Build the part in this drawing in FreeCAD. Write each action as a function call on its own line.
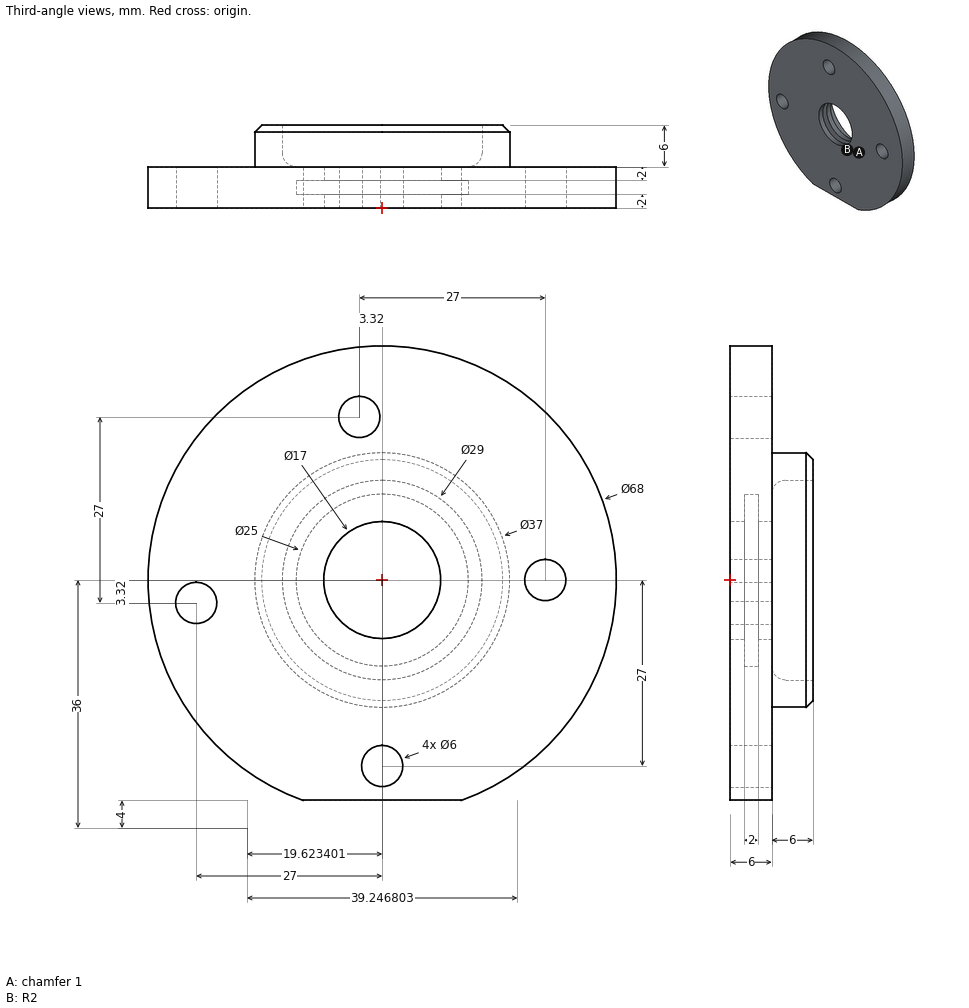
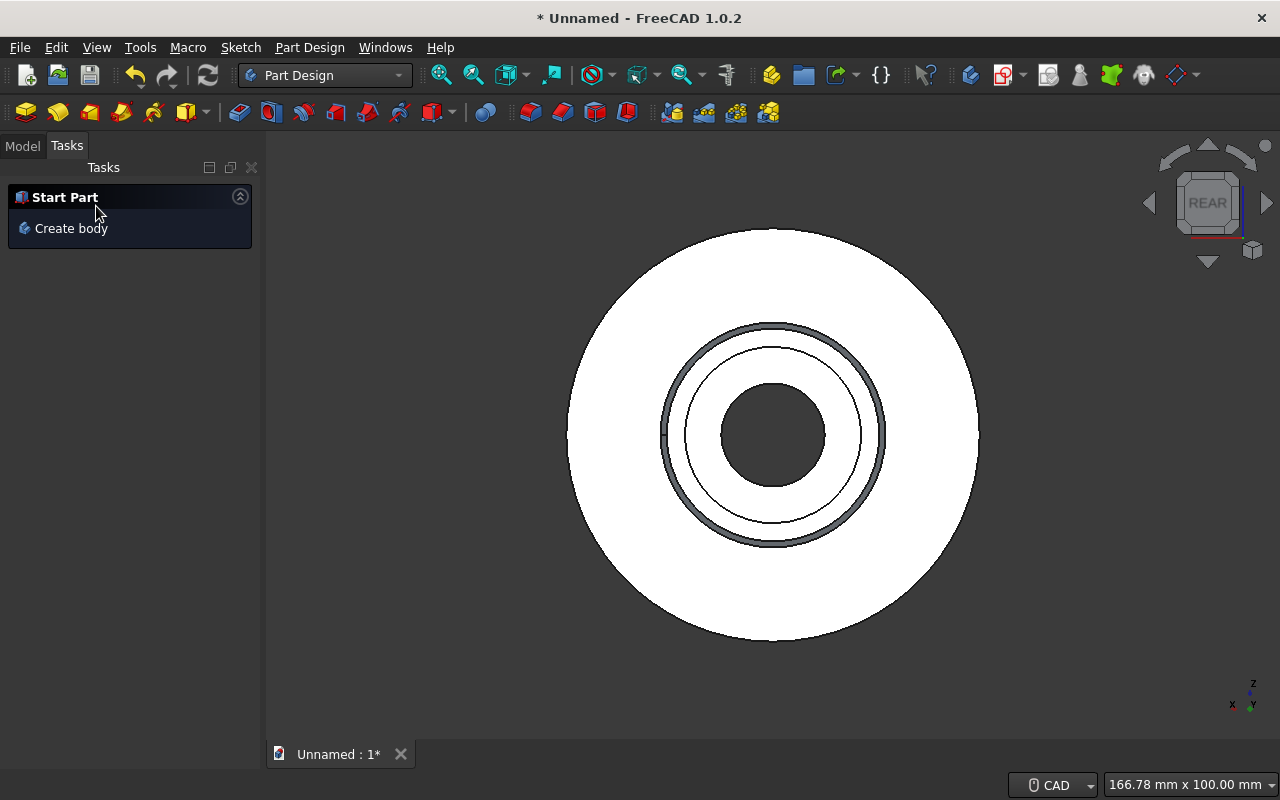
key(0)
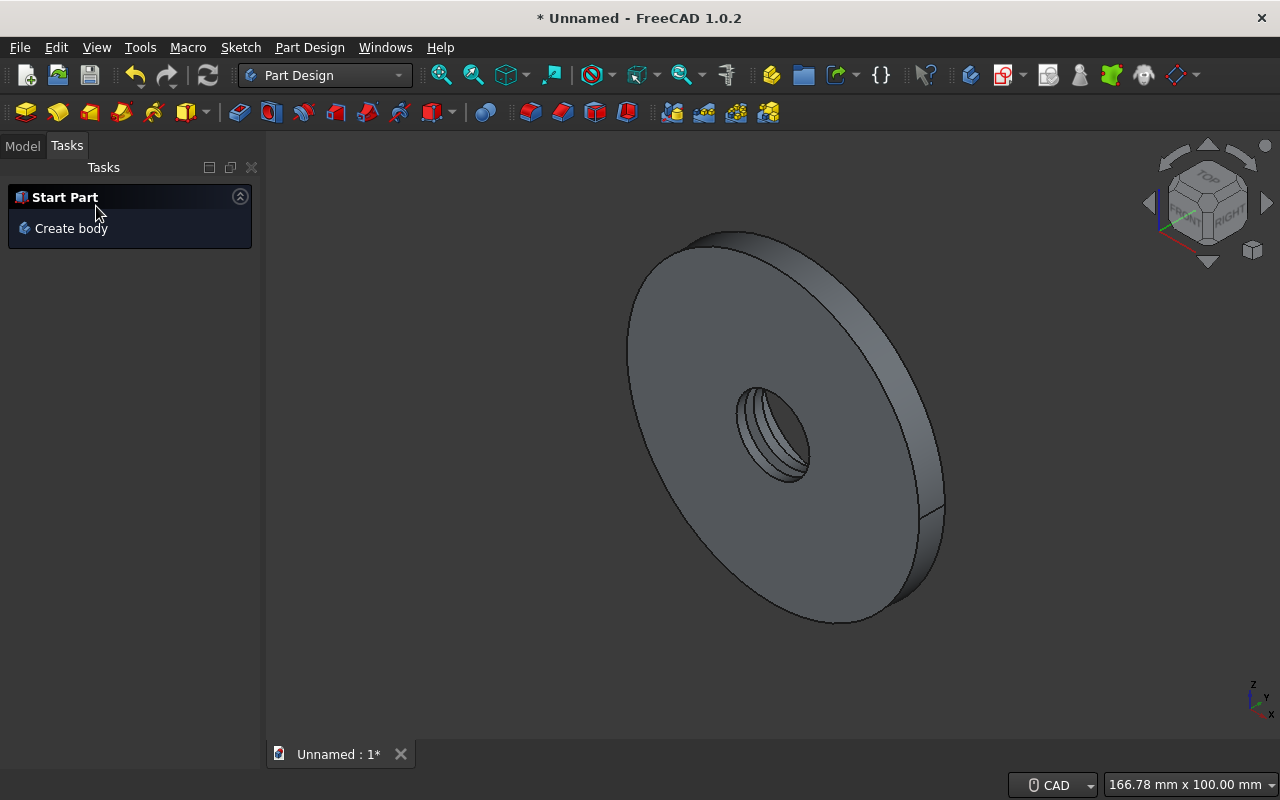
key(2)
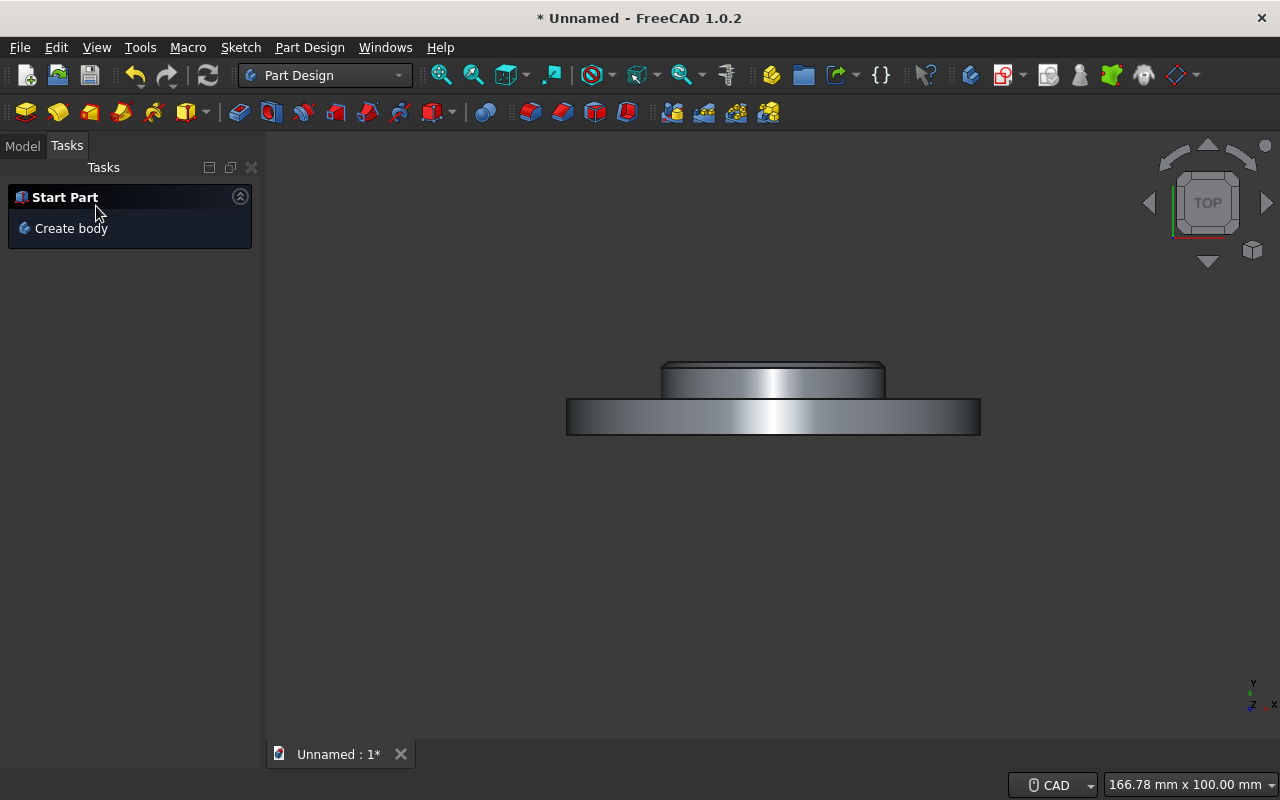
click(442, 76)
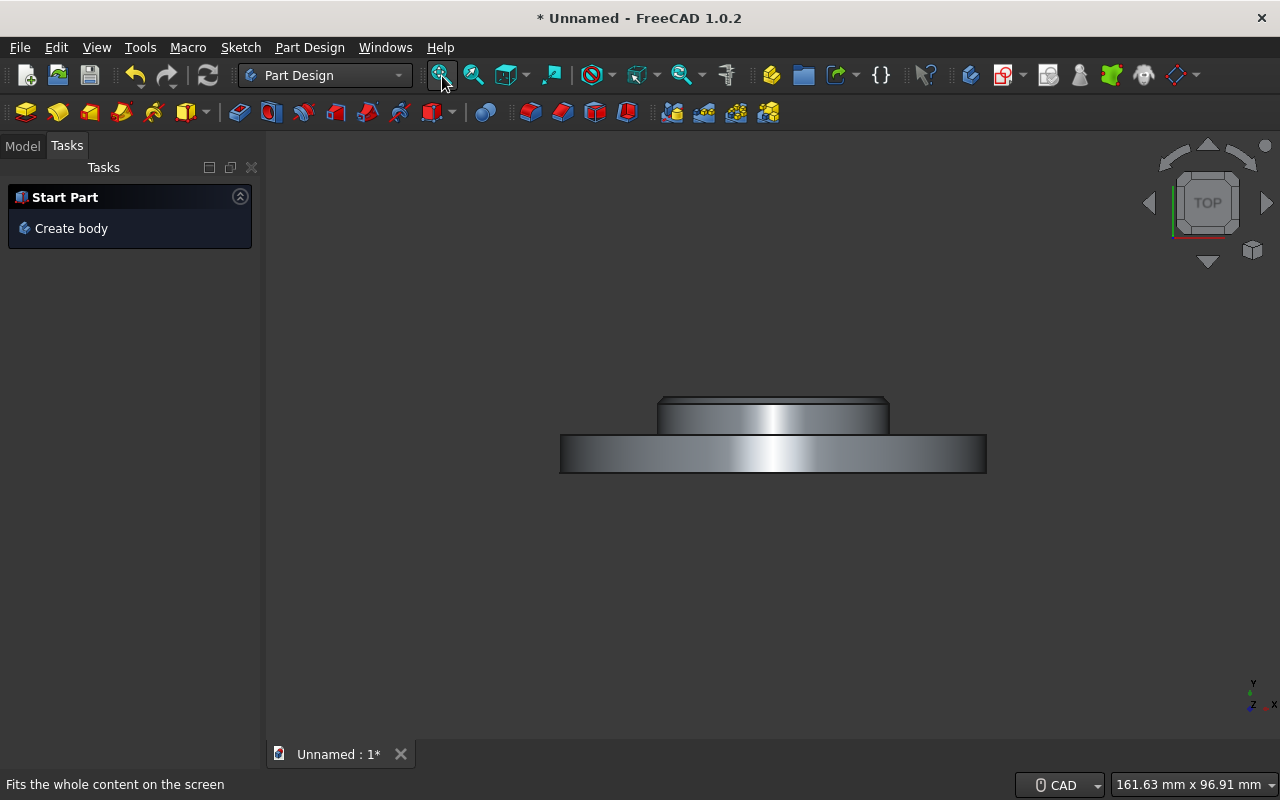
key(1)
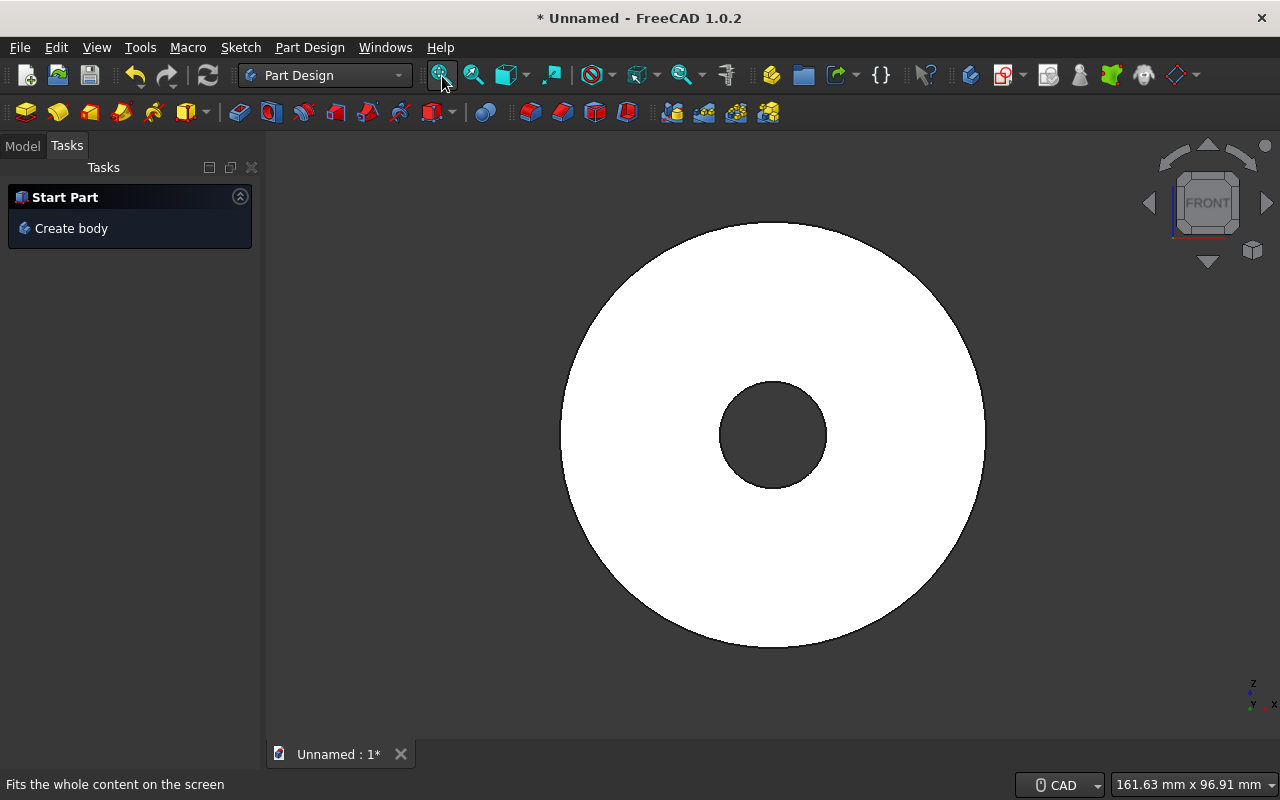
key(3)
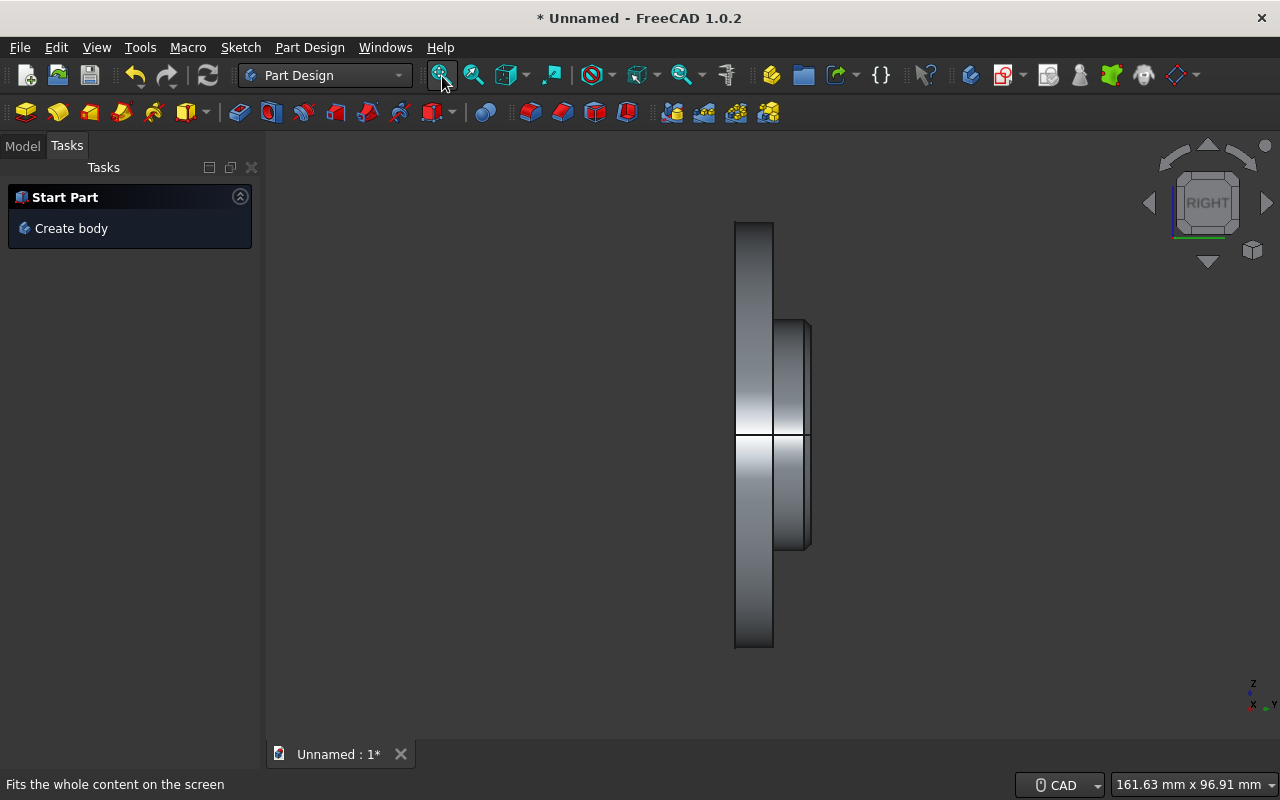
key(5)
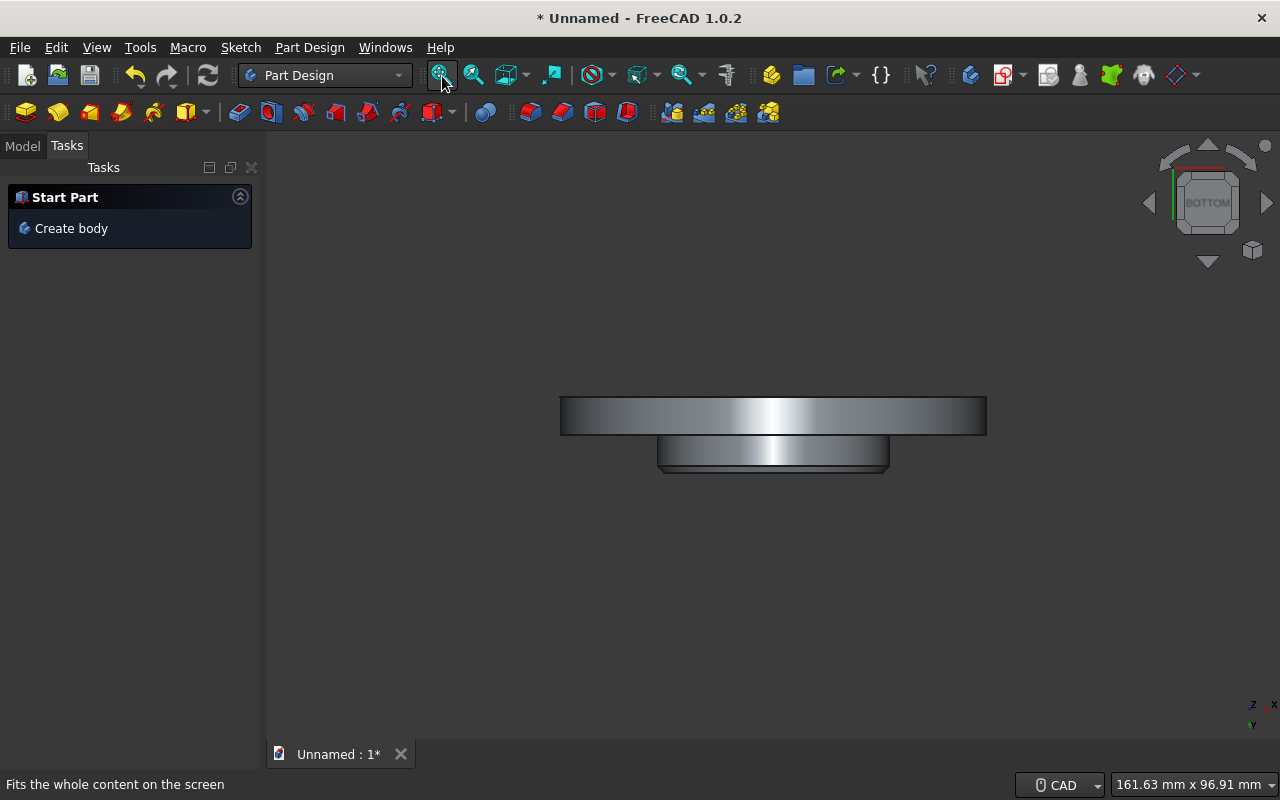
click(442, 76)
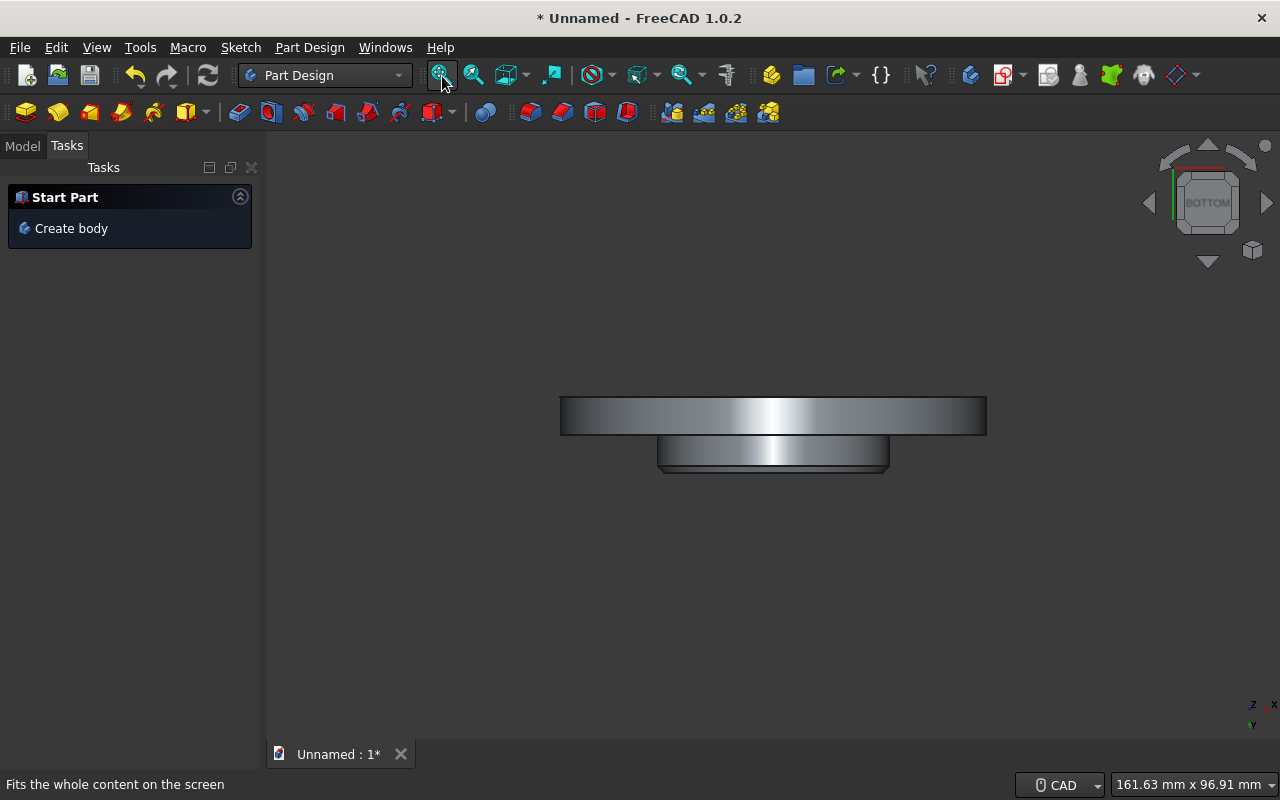
key(4)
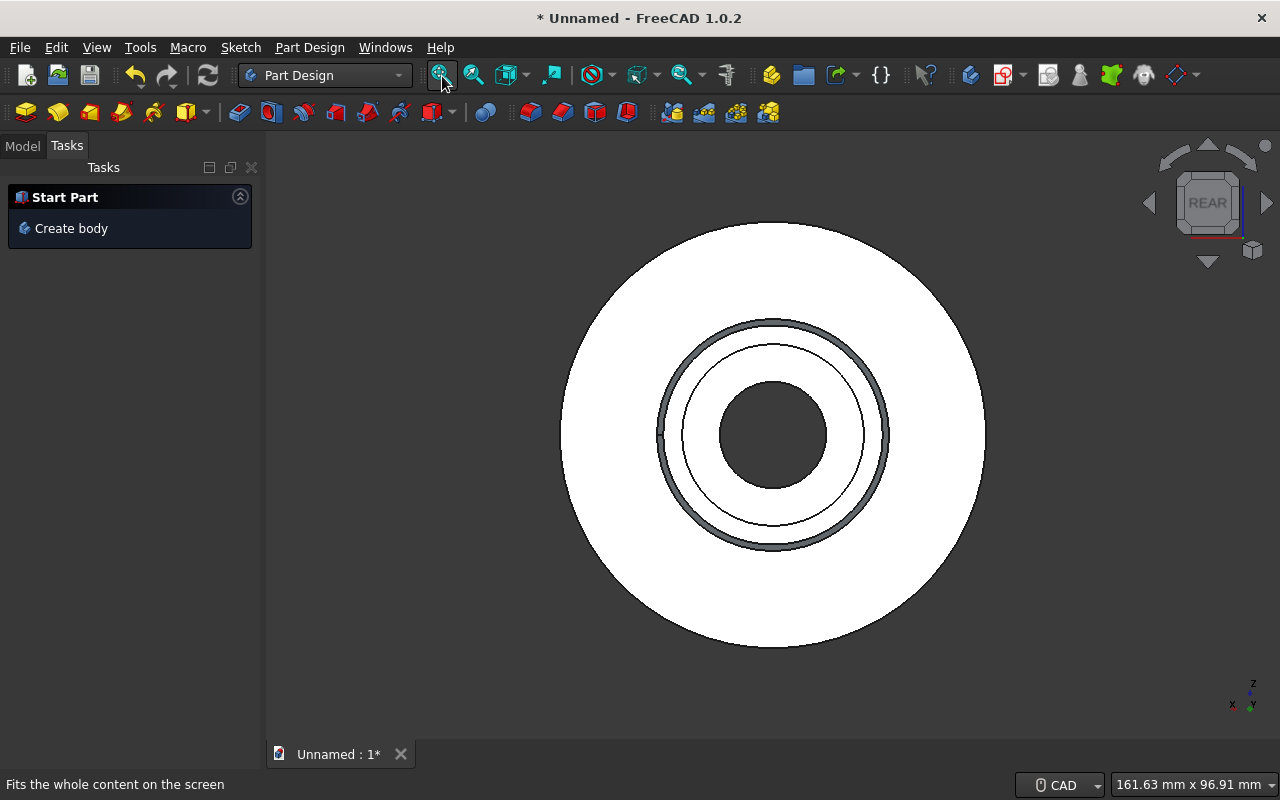
key(6)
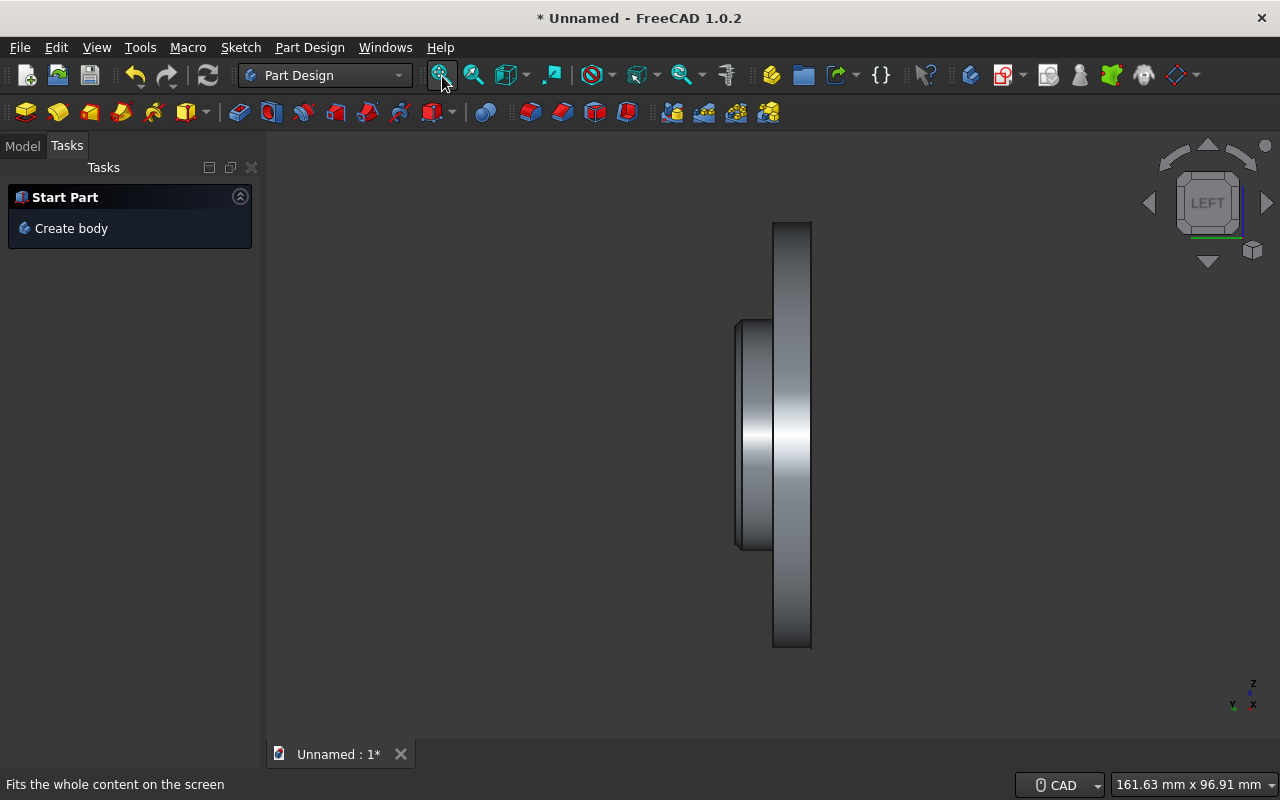
key(v)
key(3)